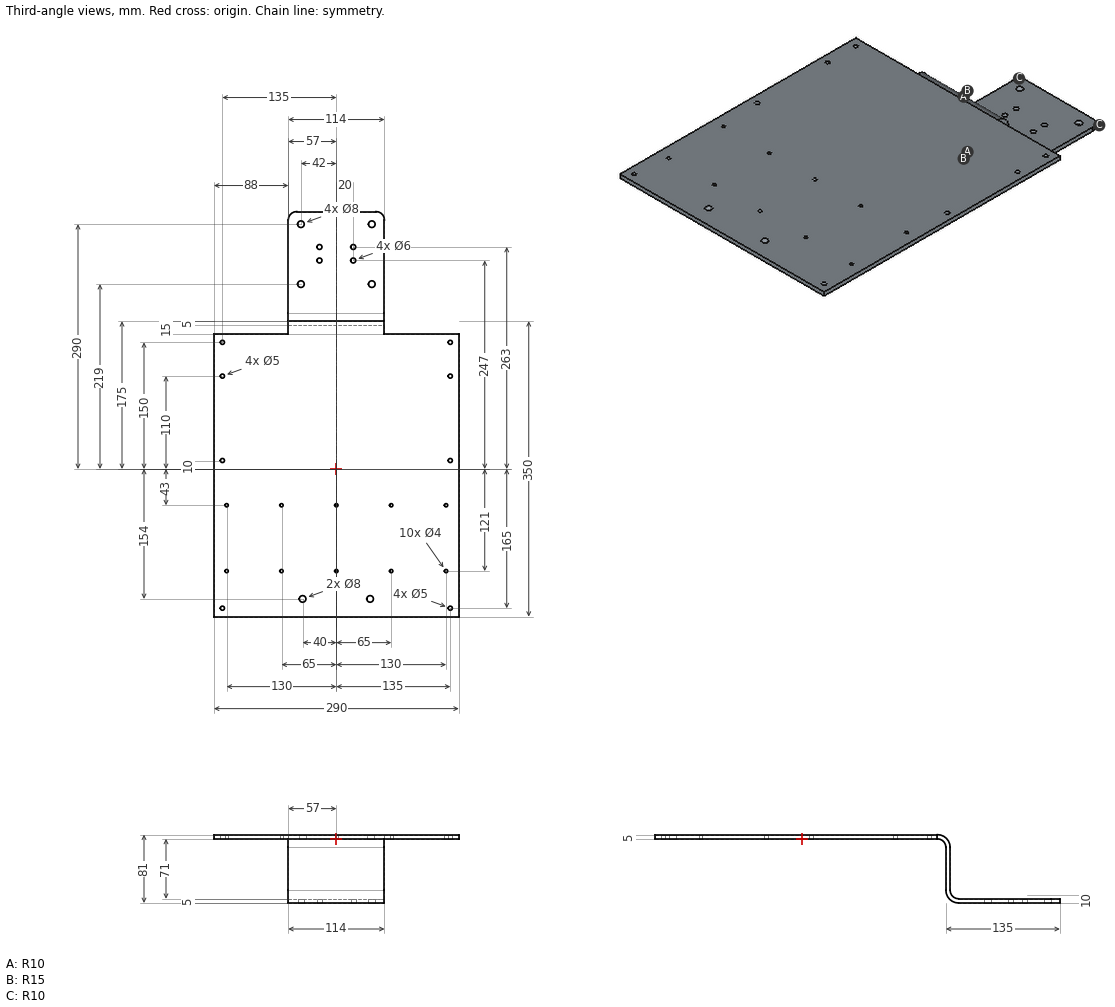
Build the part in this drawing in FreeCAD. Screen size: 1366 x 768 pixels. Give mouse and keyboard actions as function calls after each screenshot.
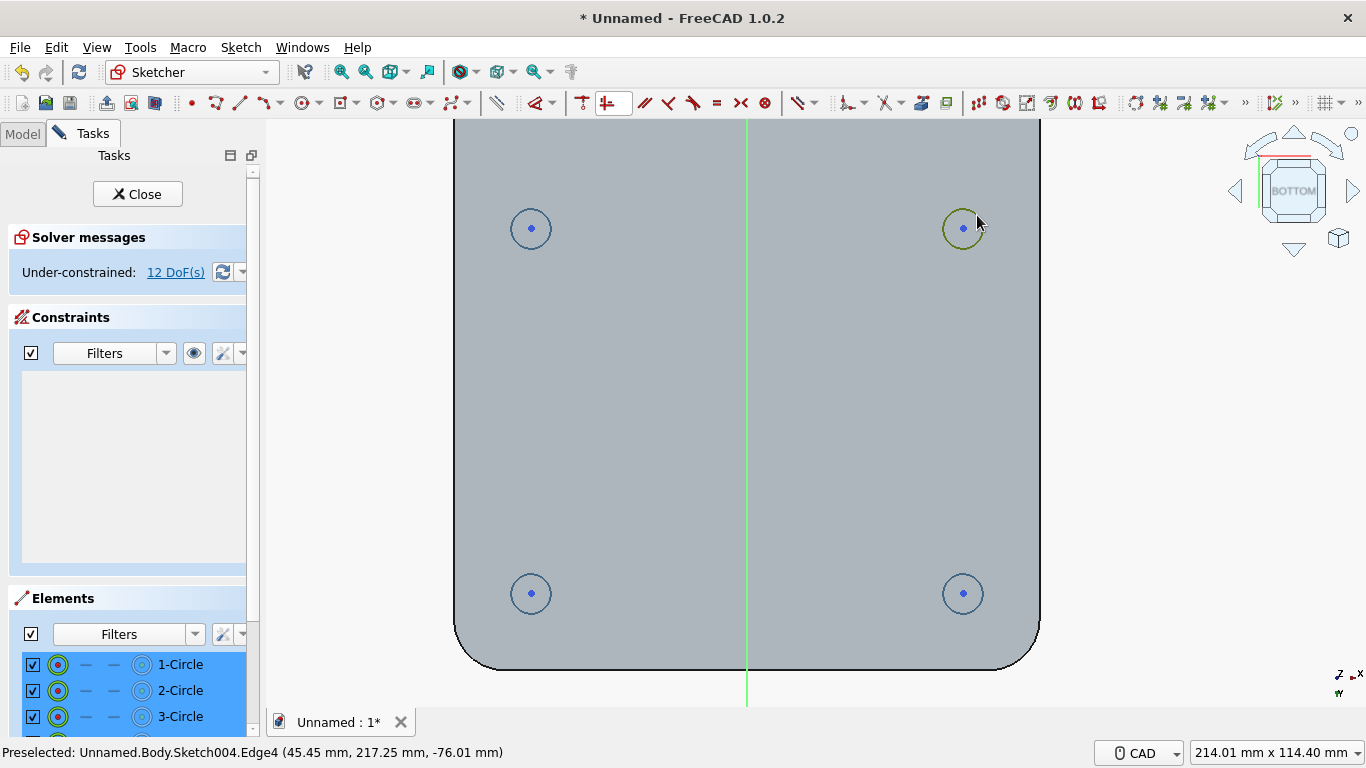
click(718, 104)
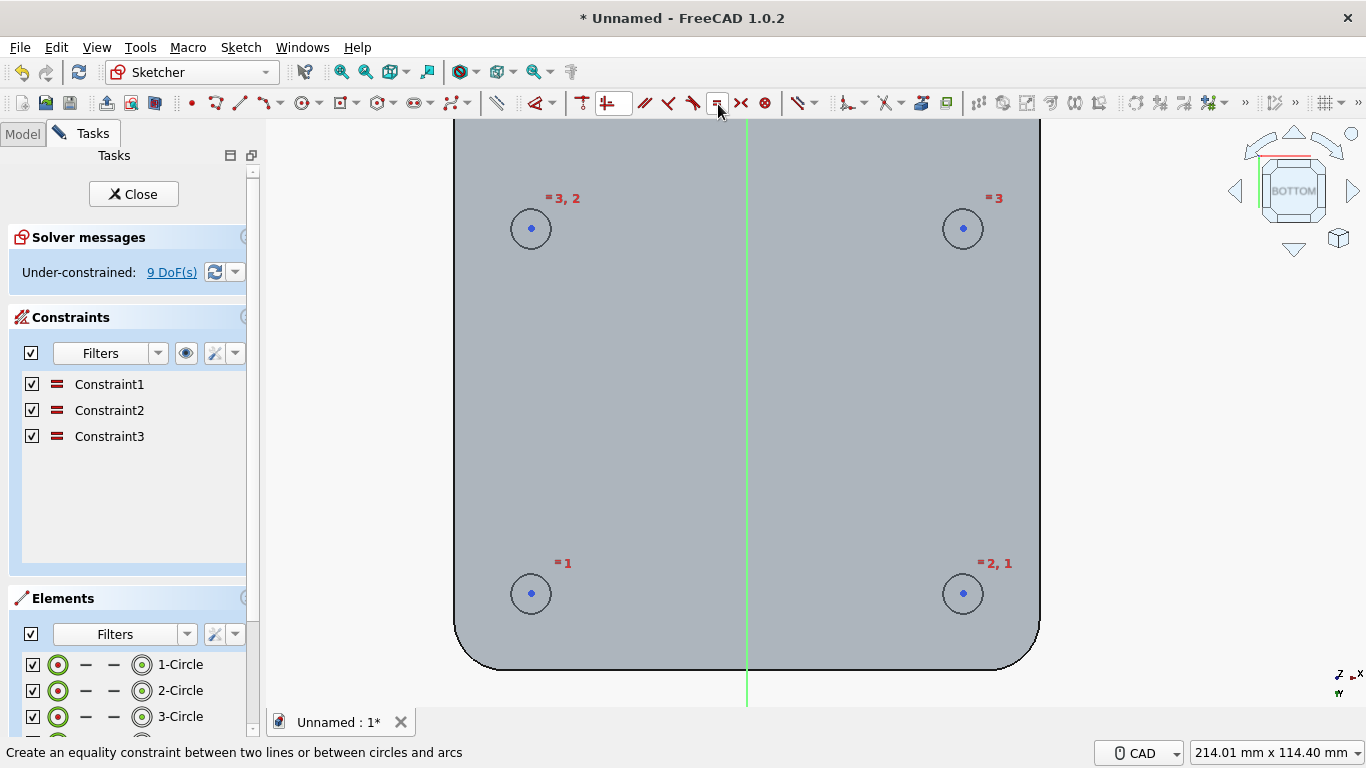
click(531, 594)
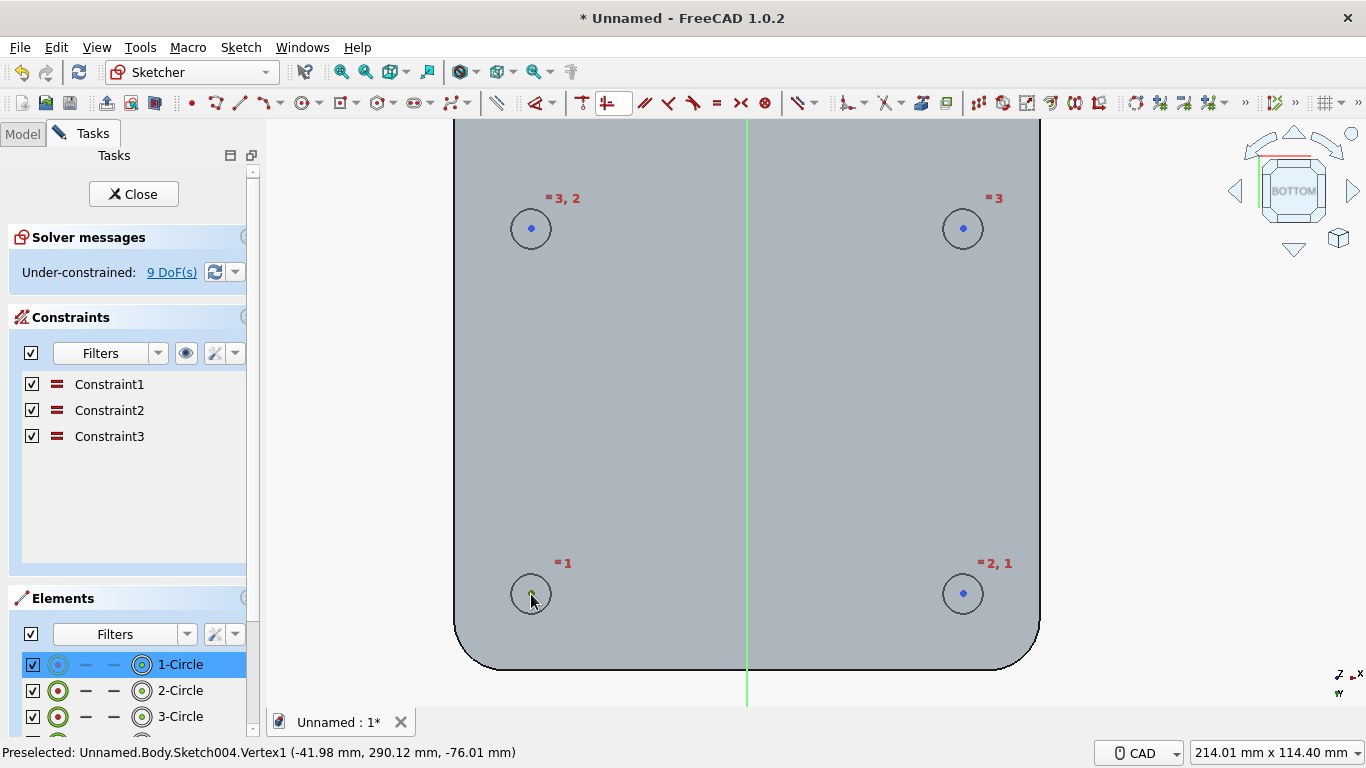
click(963, 594)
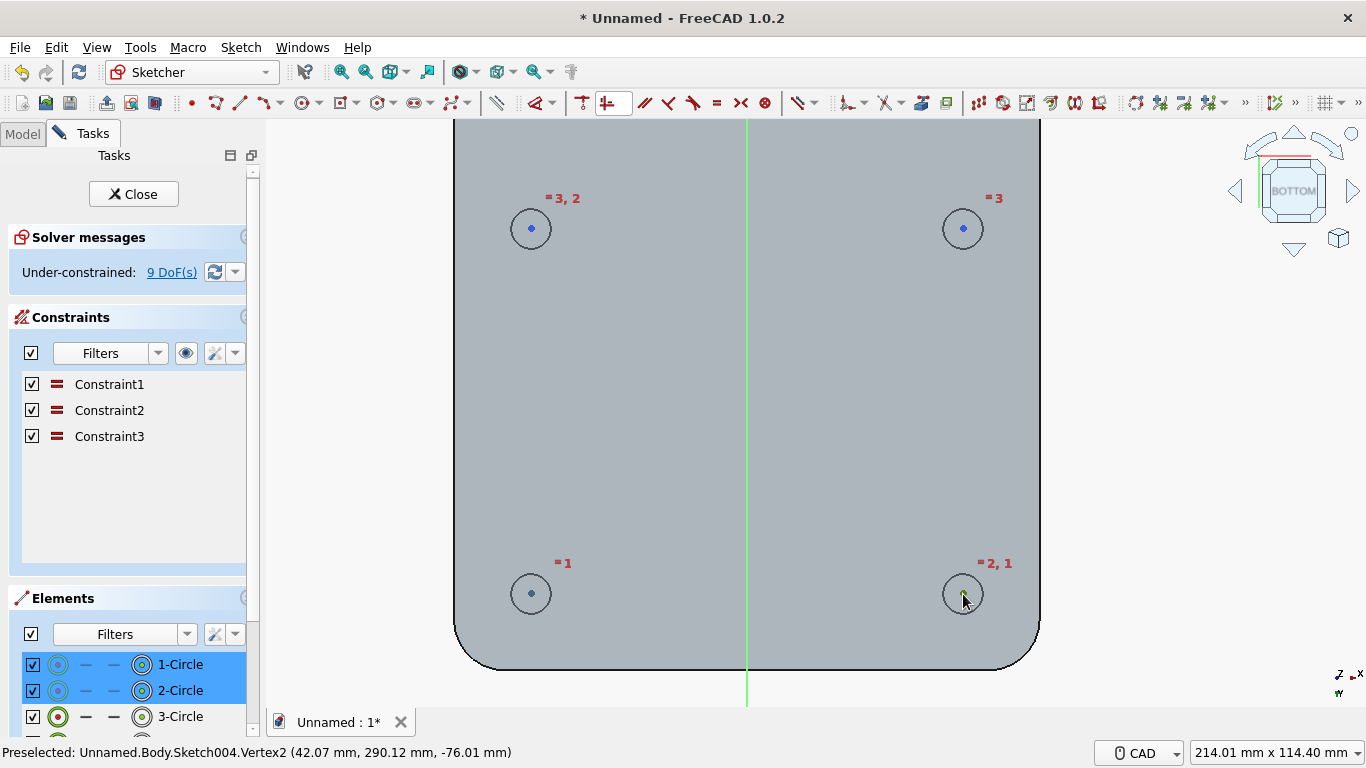
click(747, 641)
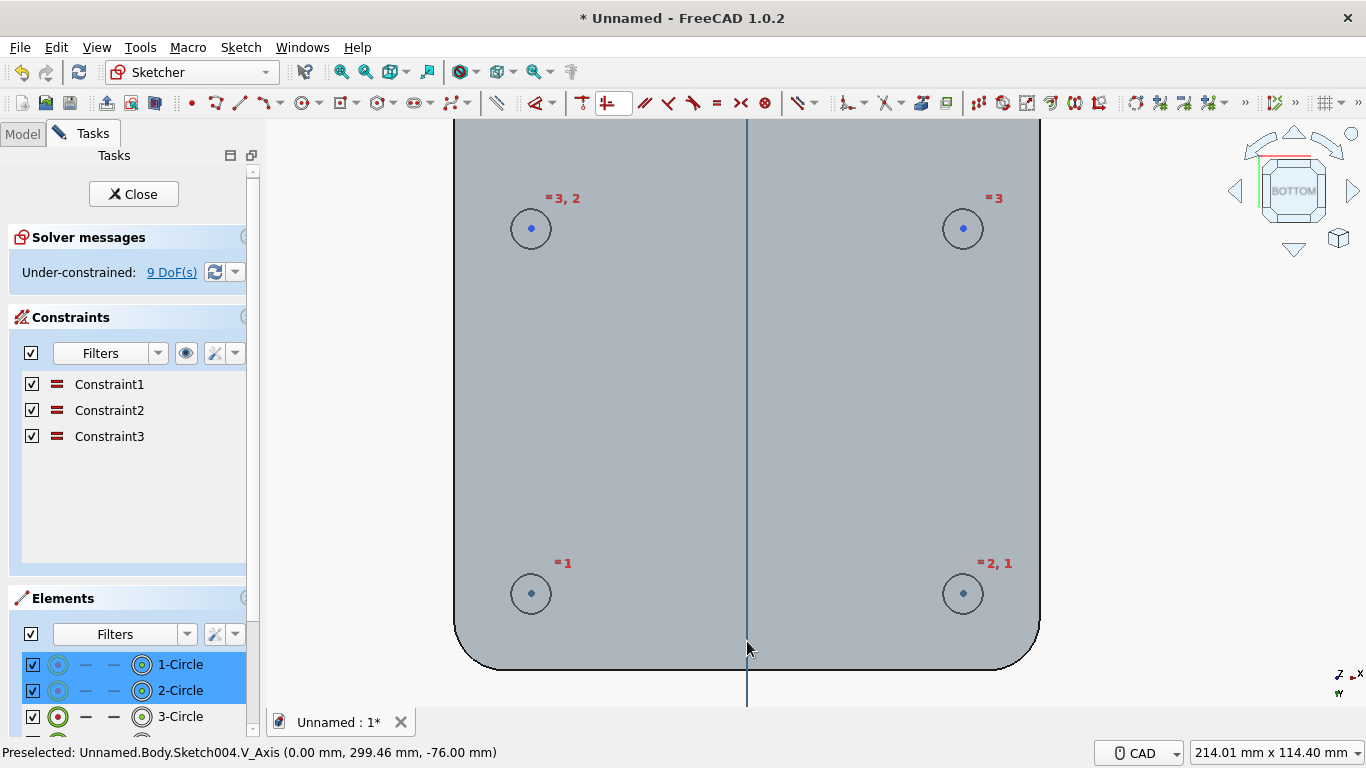
click(742, 104)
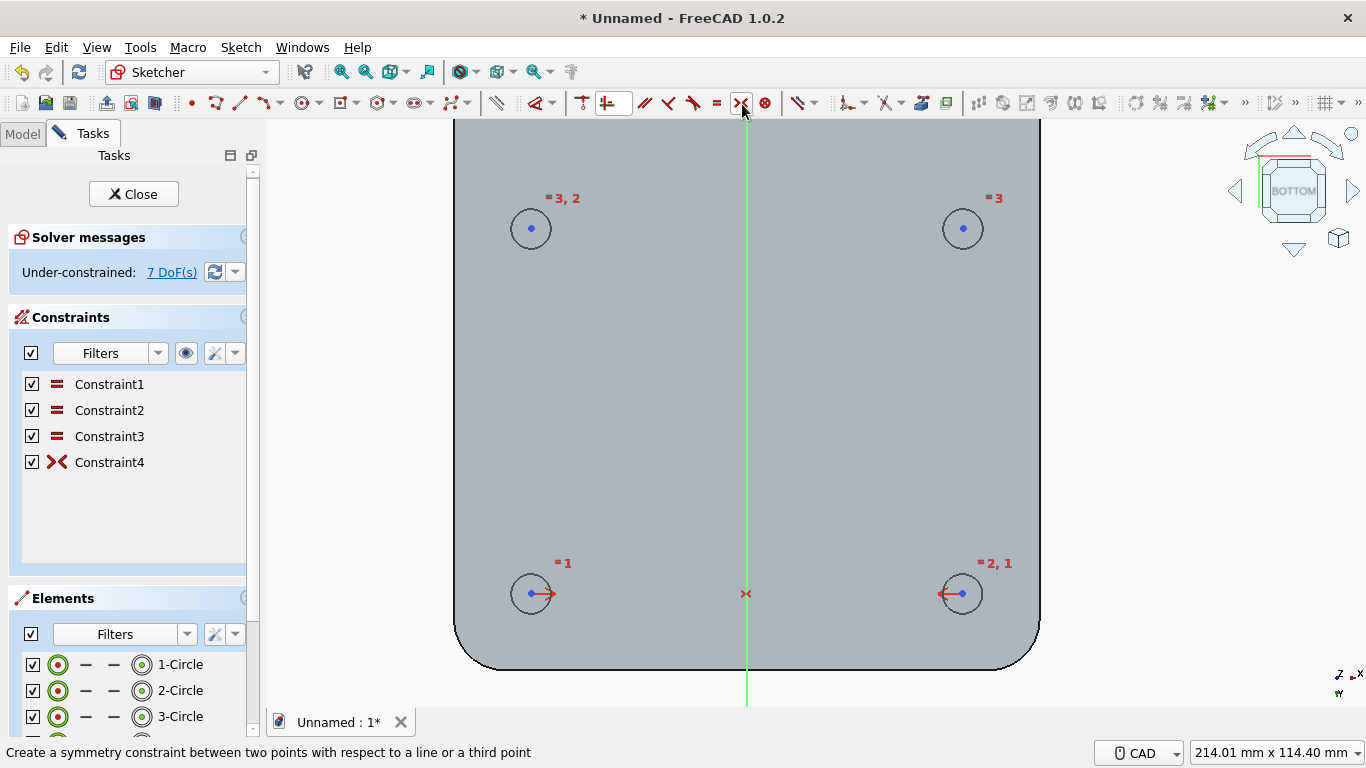
click(531, 229)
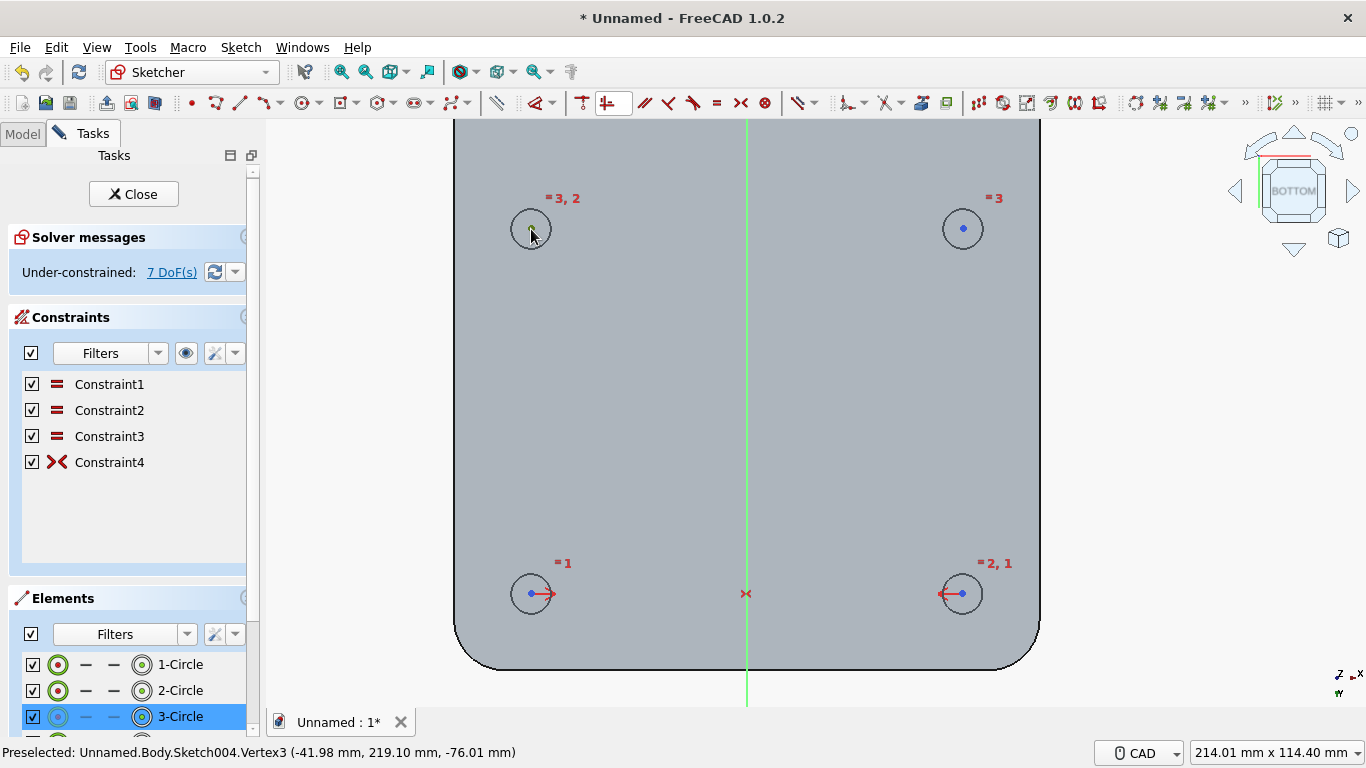
click(963, 229)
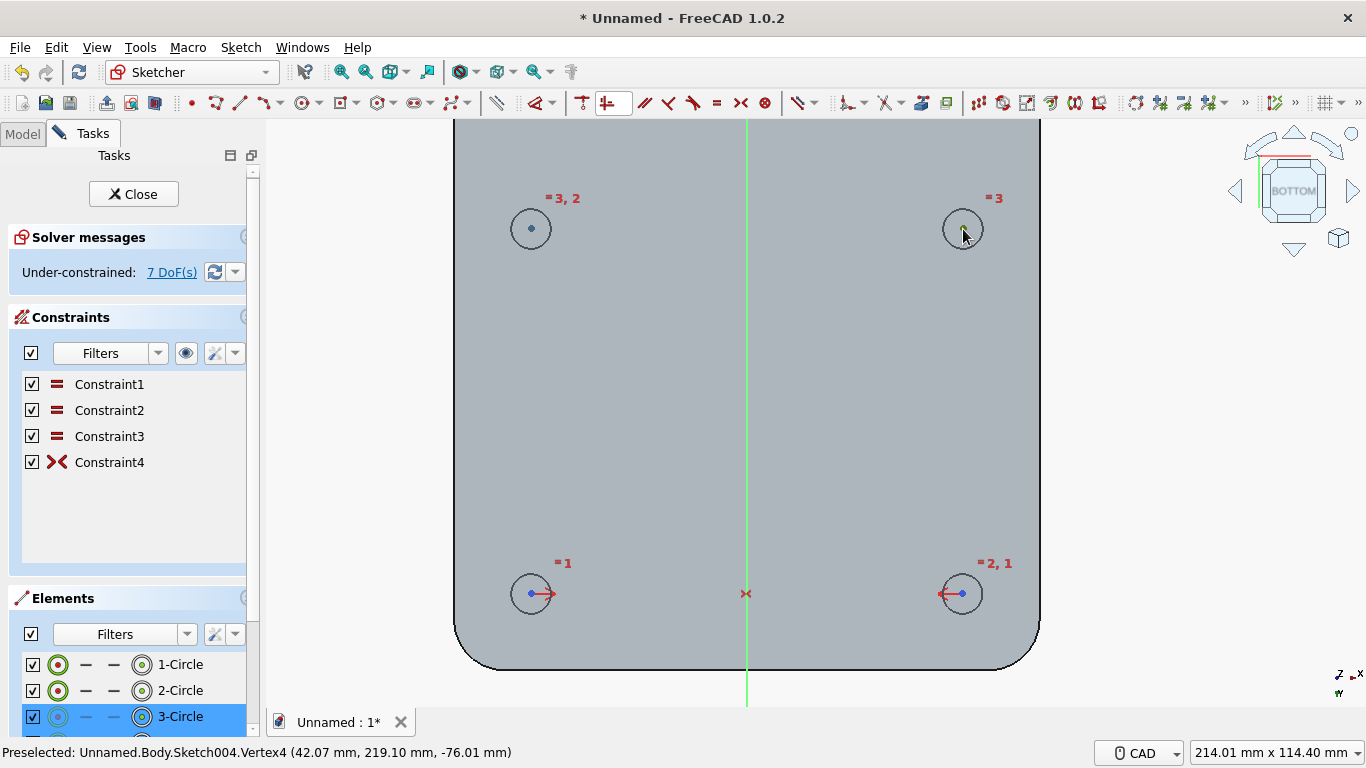
click(747, 641)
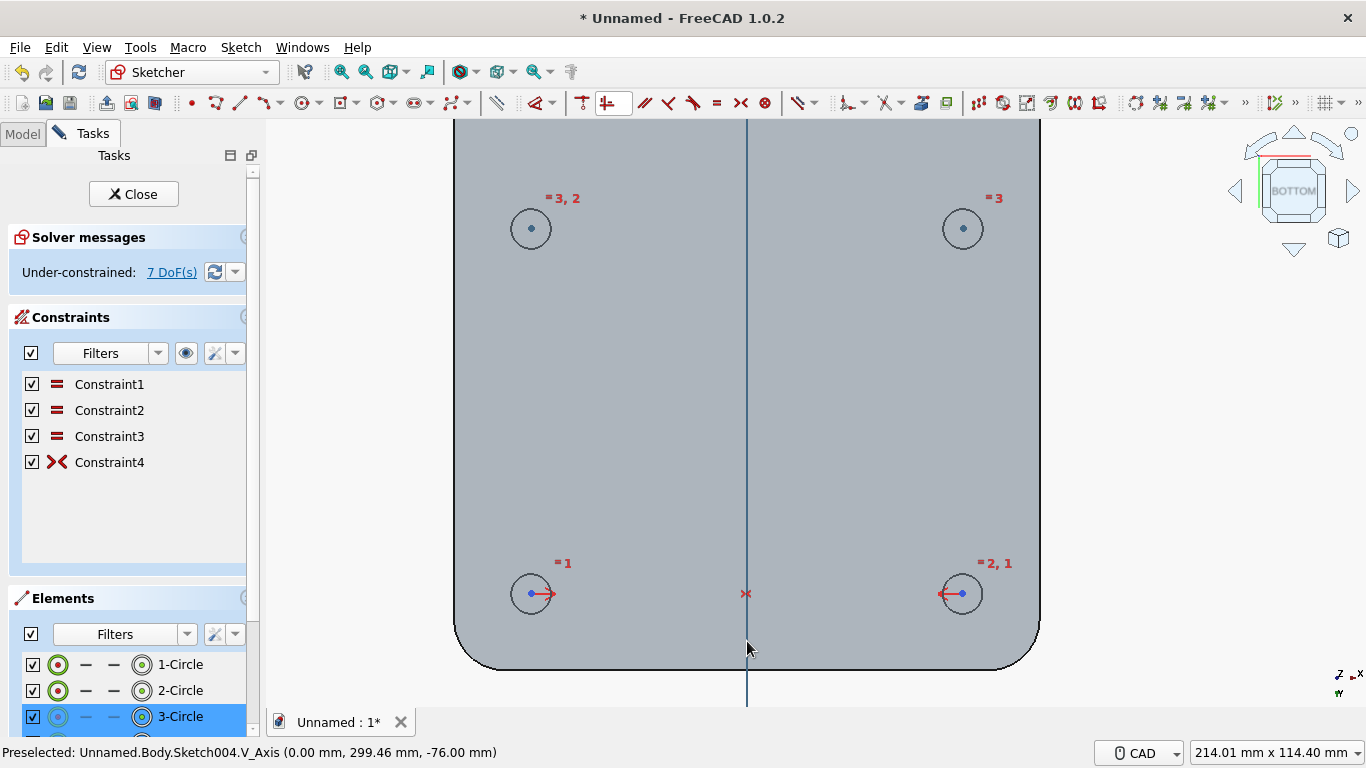
click(742, 104)